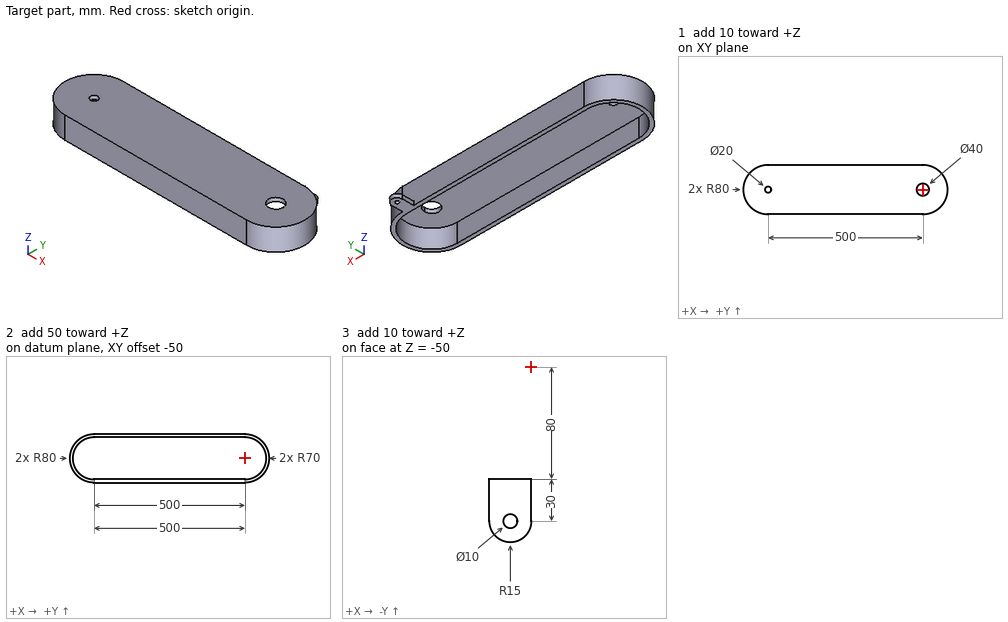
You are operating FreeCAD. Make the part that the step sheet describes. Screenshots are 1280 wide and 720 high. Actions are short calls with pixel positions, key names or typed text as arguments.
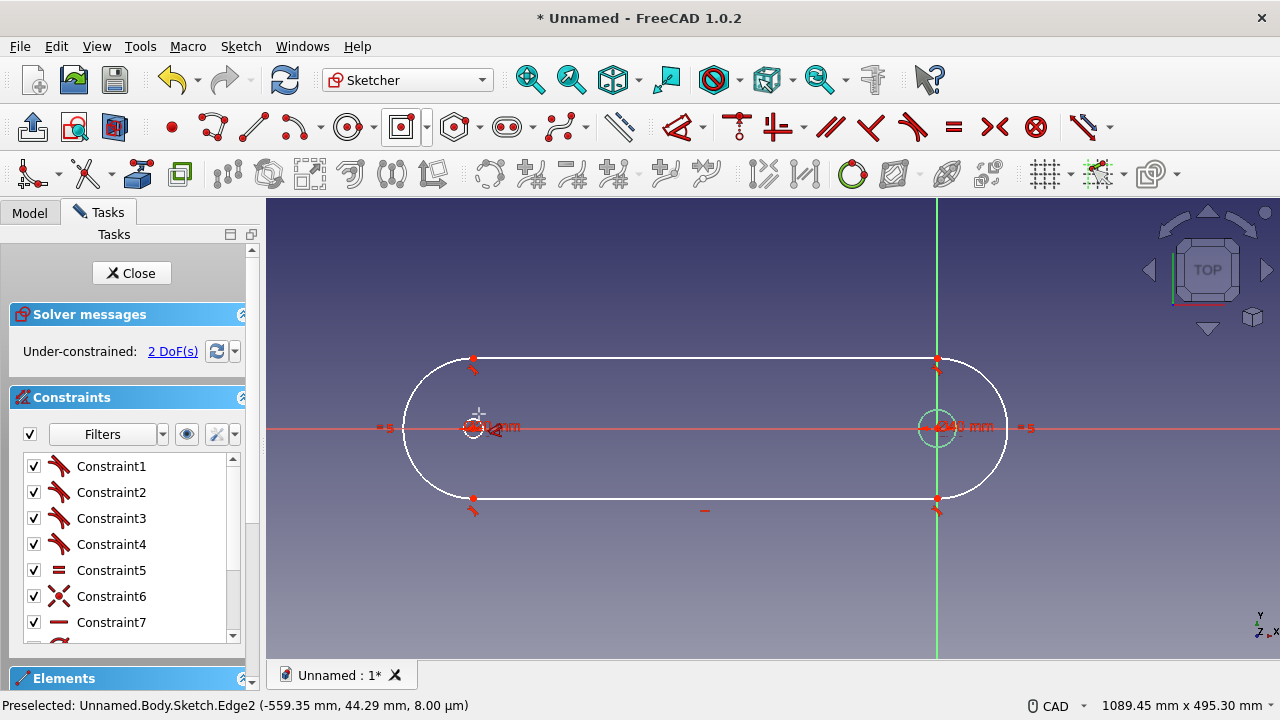
click(994, 470)
click(1020, 489)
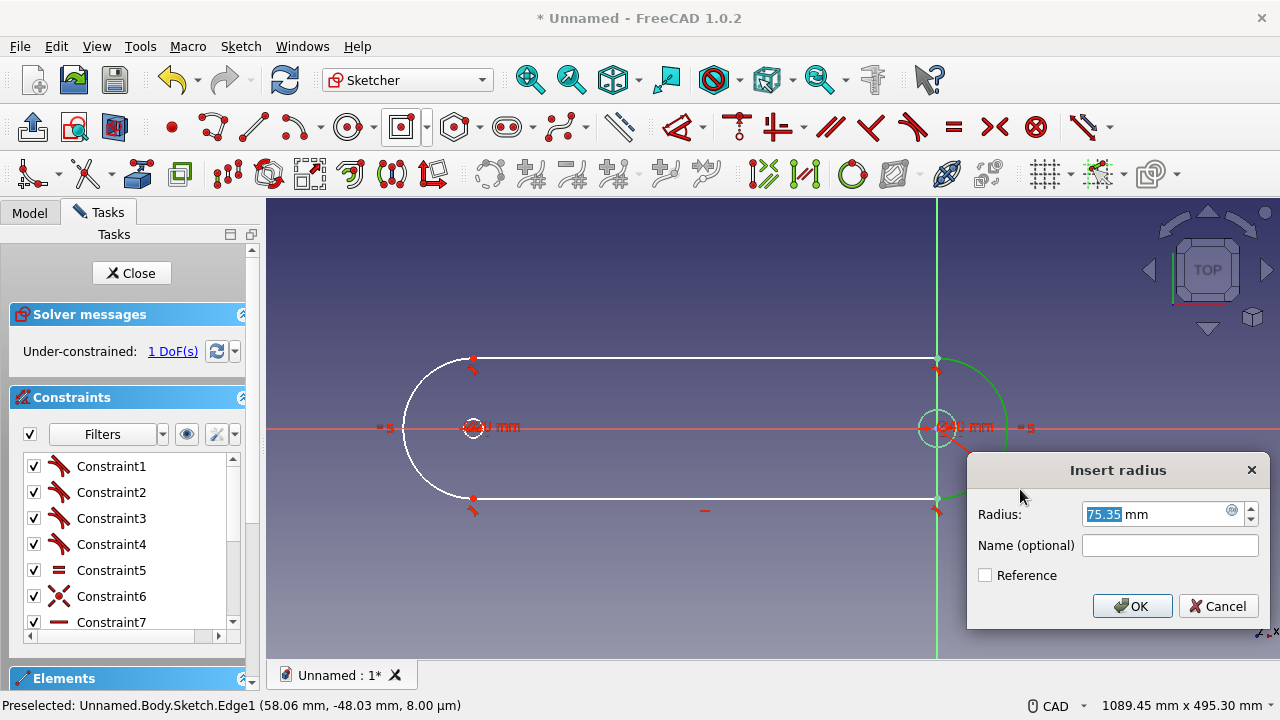
text(80)
key(Return)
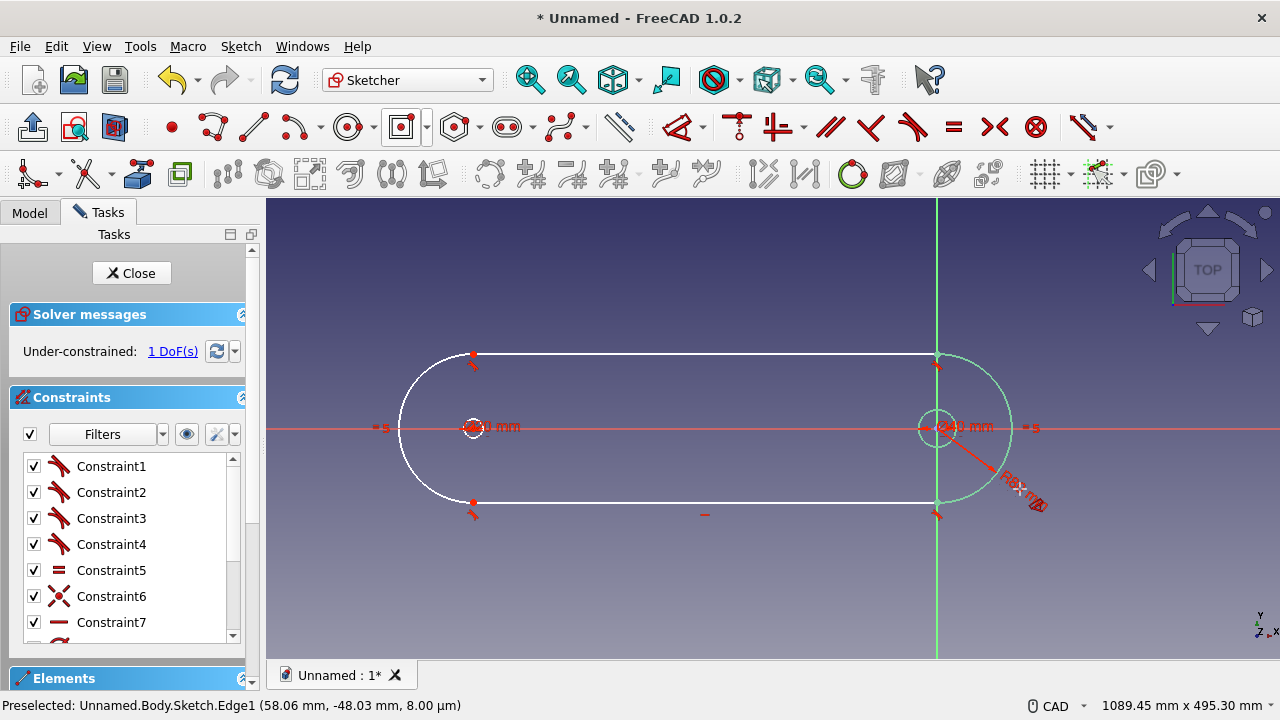
click(798, 503)
click(705, 537)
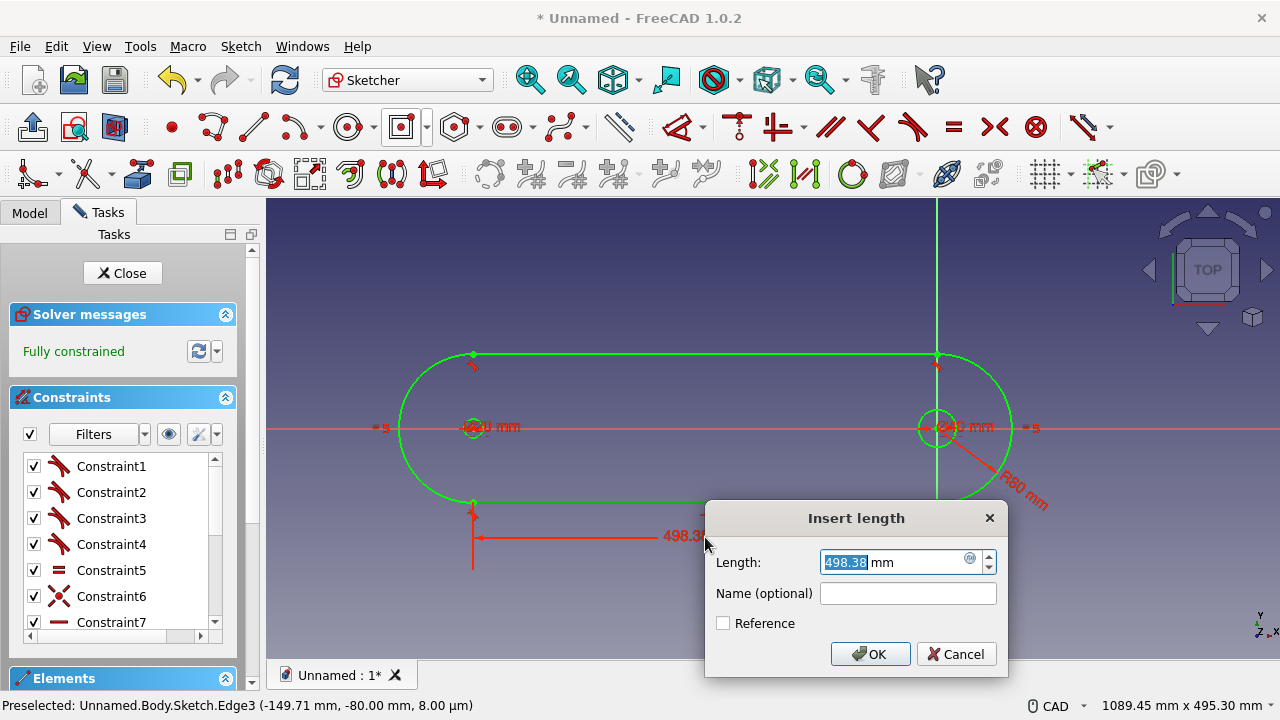
text(500)
key(Return)
key(Escape)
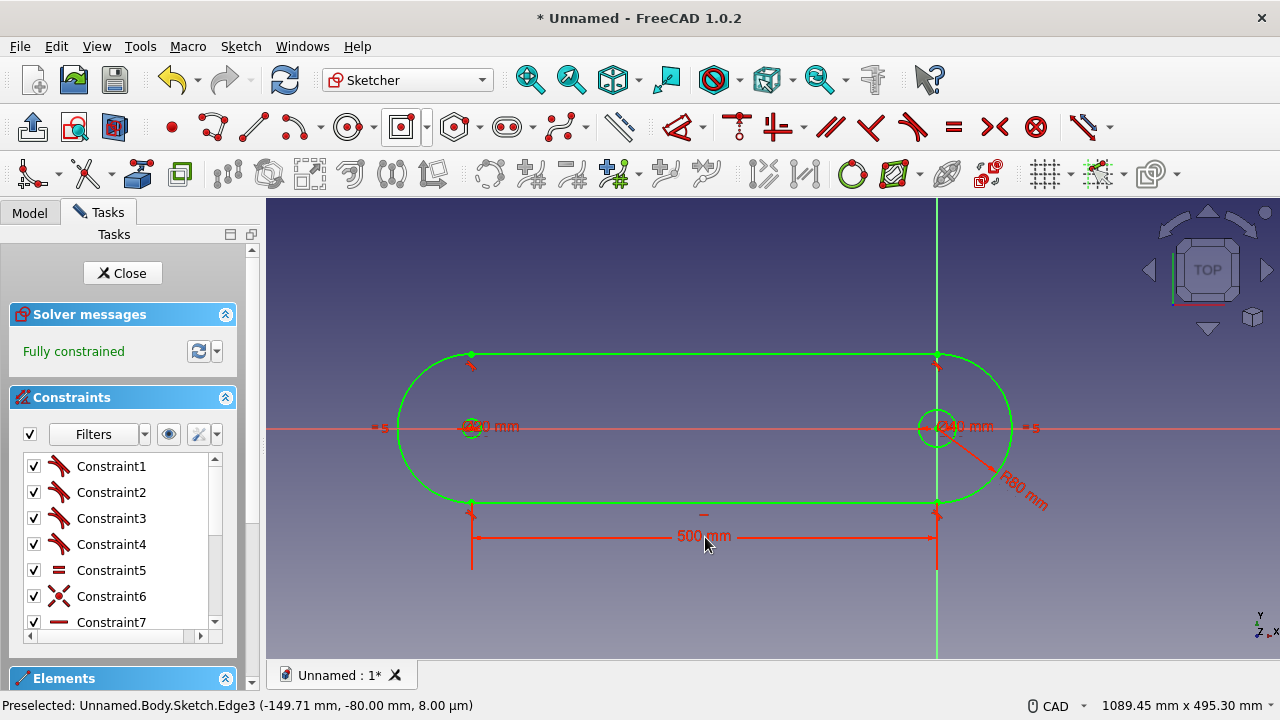
click(123, 273)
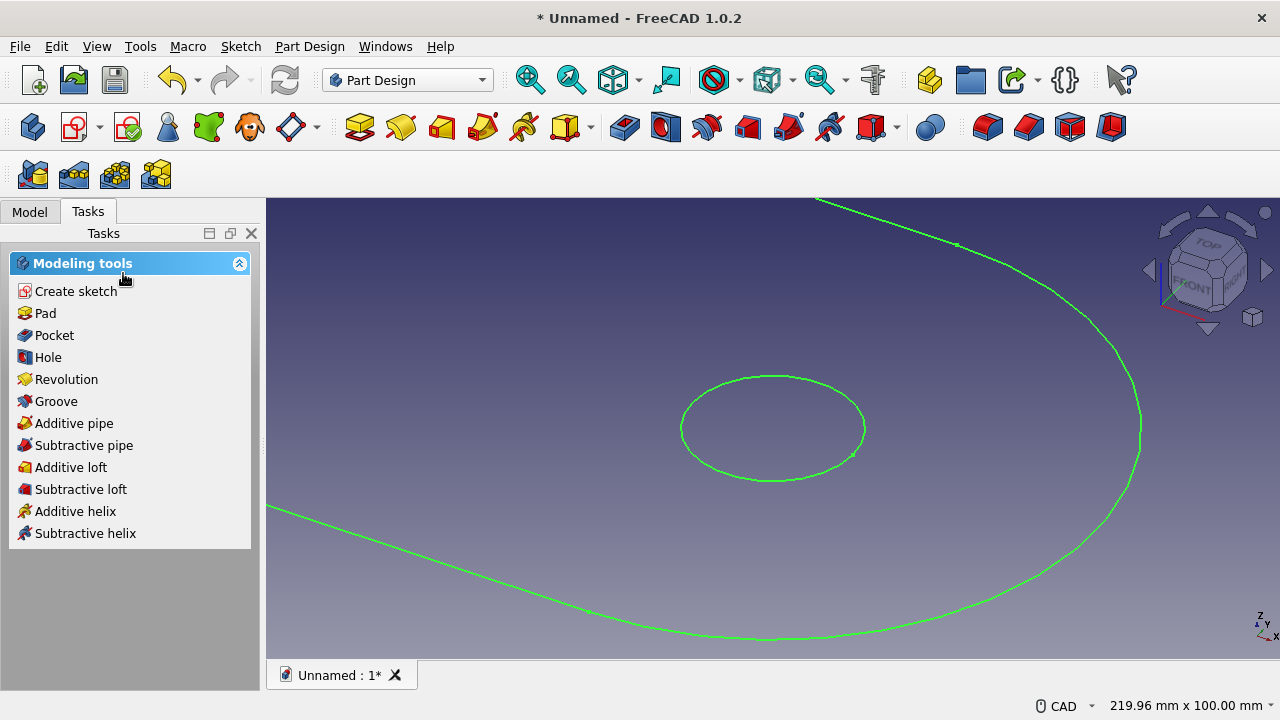
click(360, 128)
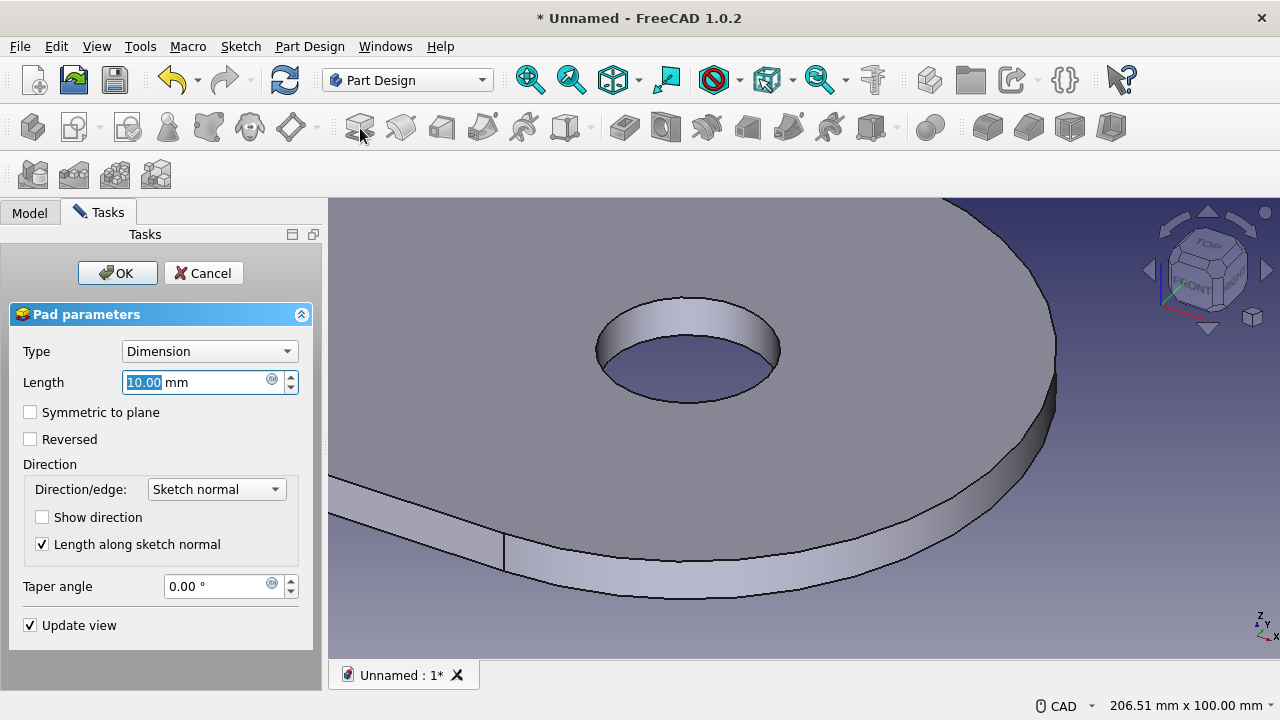
text(10)
key(Tab)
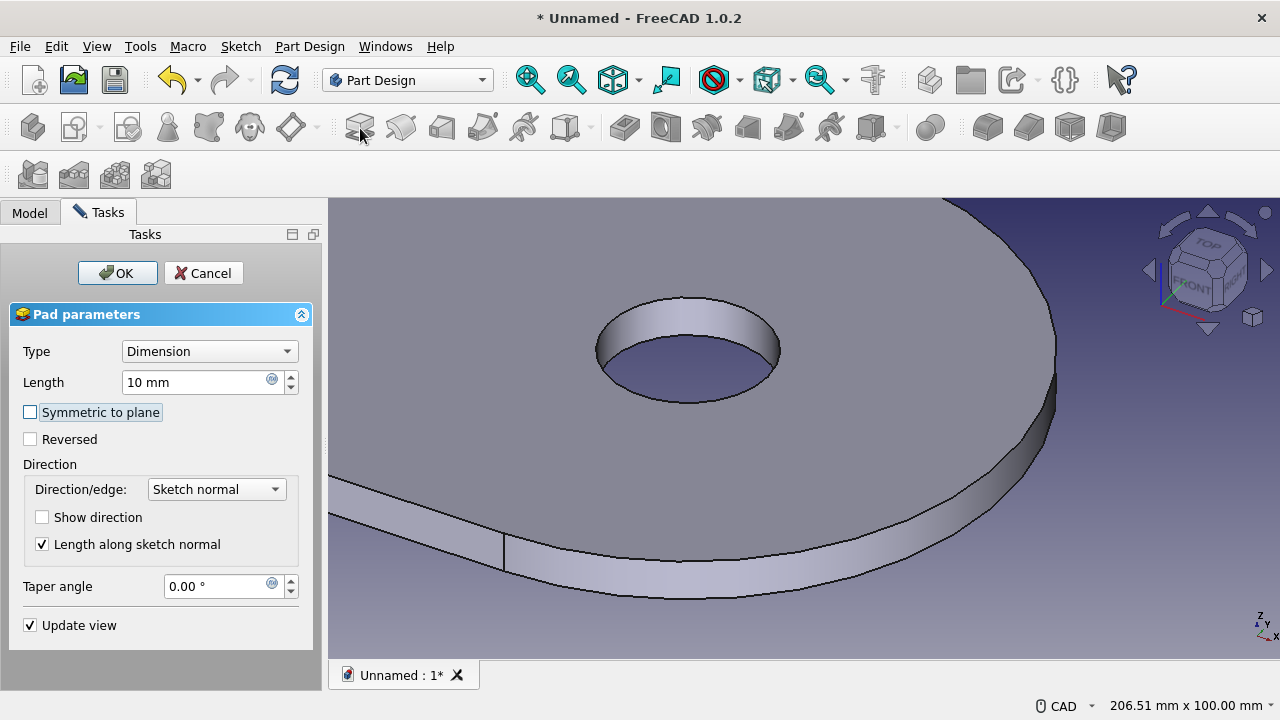
click(118, 273)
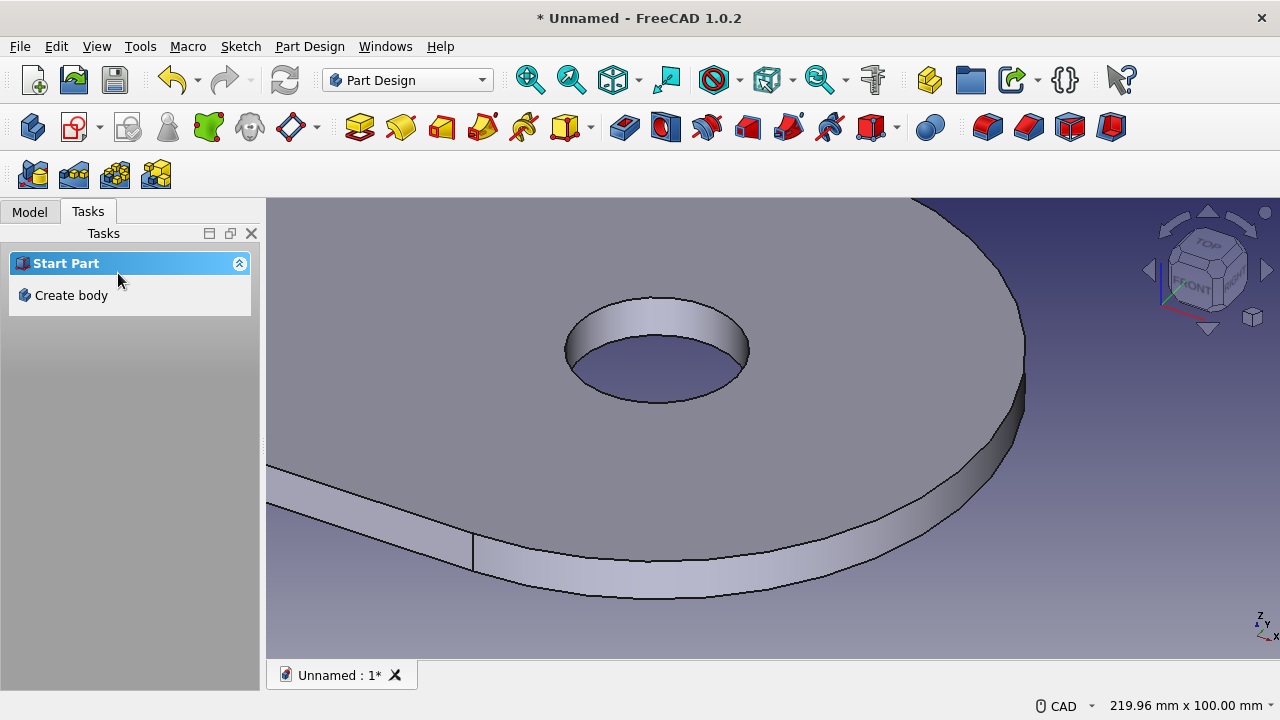
click(531, 80)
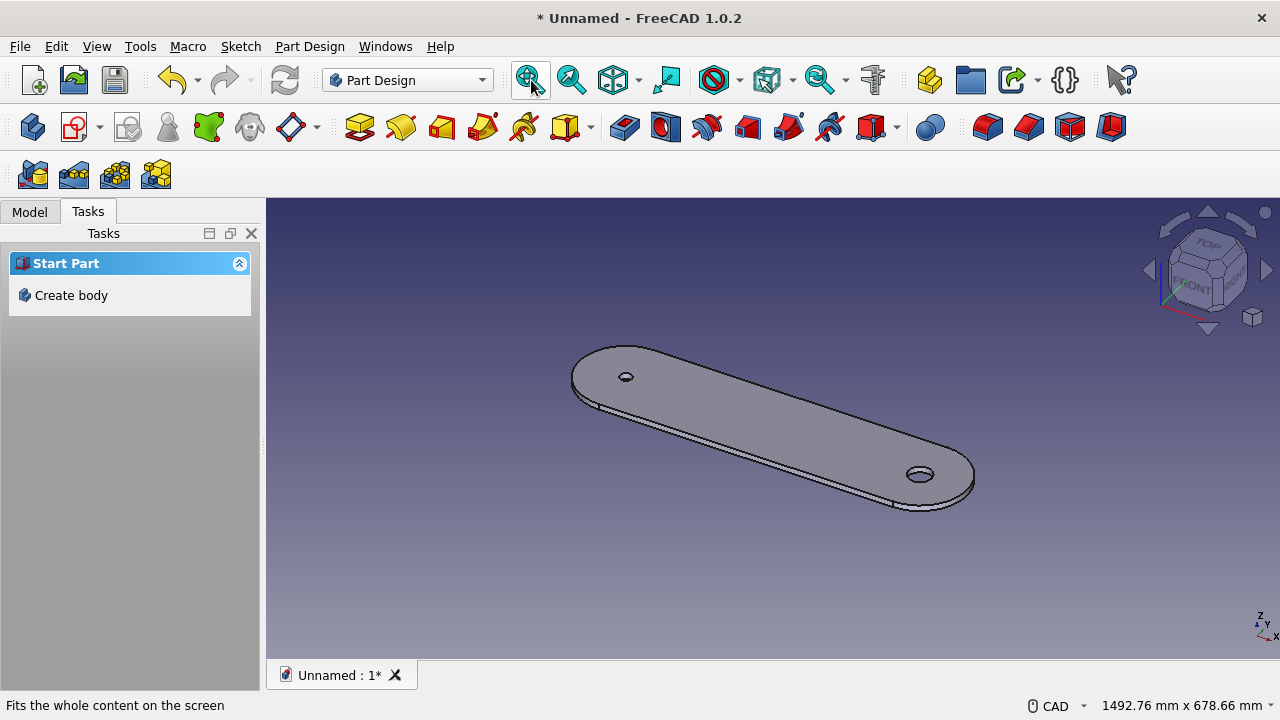
click(30, 212)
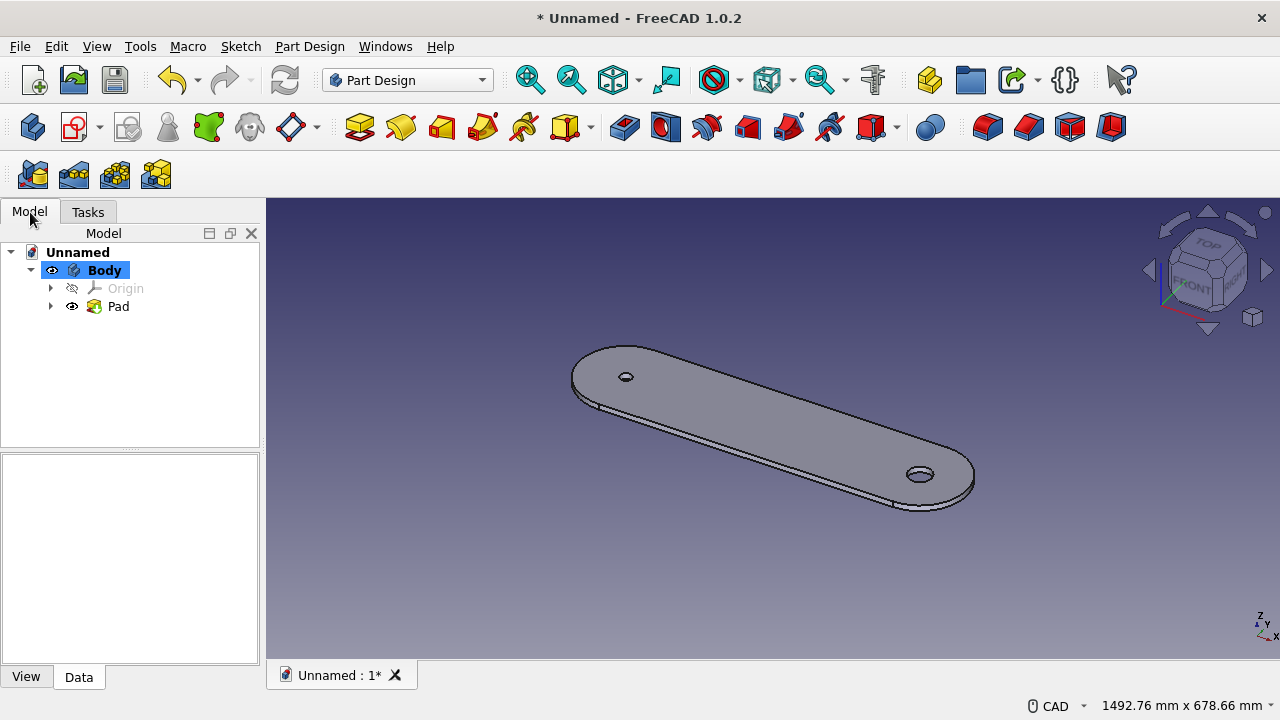
click(51, 288)